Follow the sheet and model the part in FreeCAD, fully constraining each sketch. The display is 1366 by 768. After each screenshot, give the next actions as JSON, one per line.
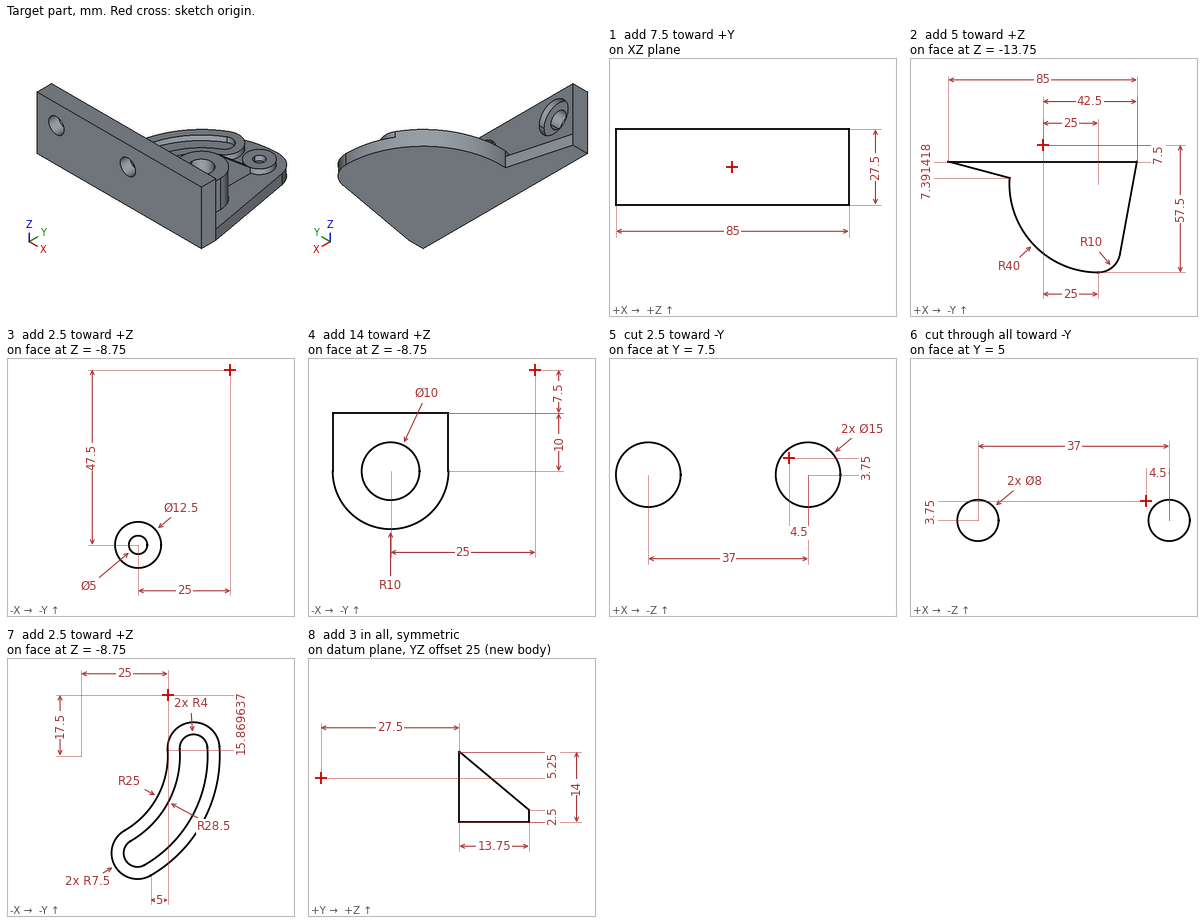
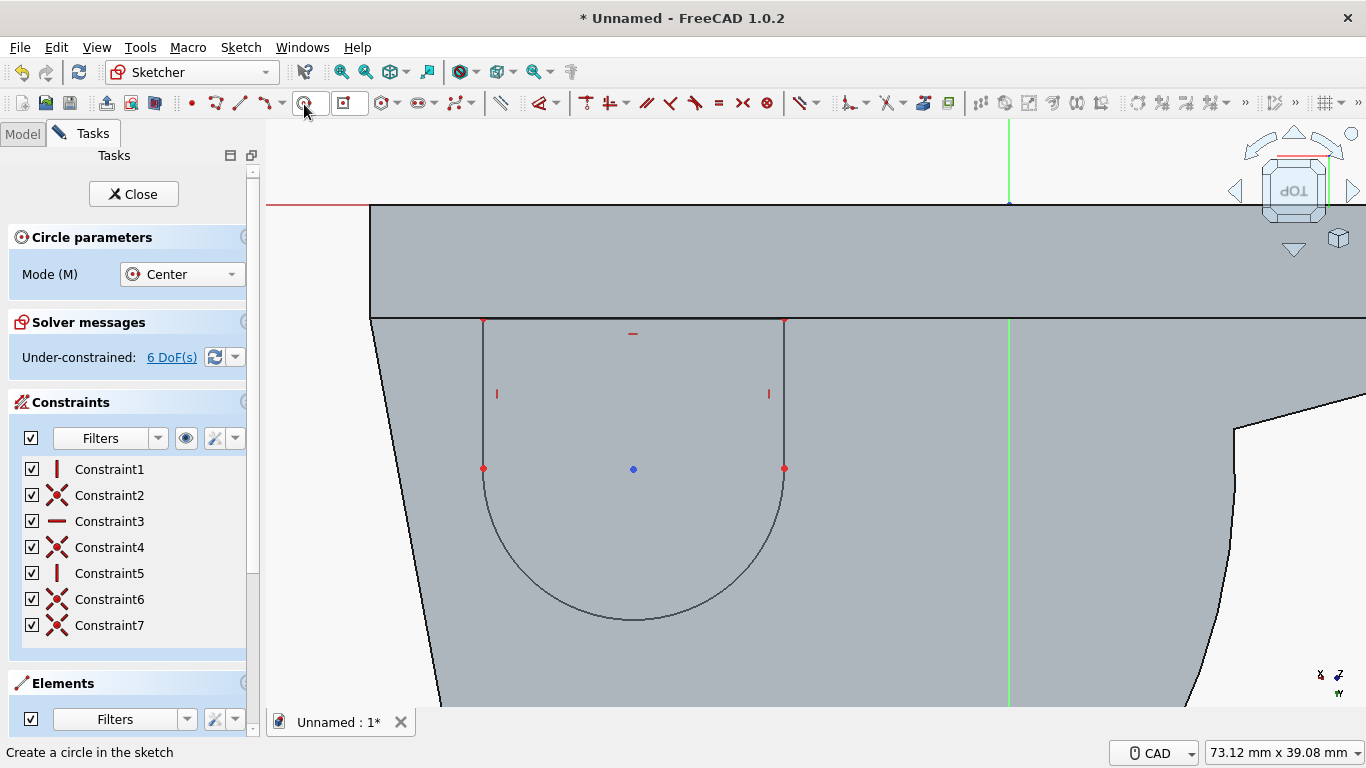
{"action": "left_click", "coordinate": [633, 468]}
{"action": "mouse_move", "coordinate": [687, 415]}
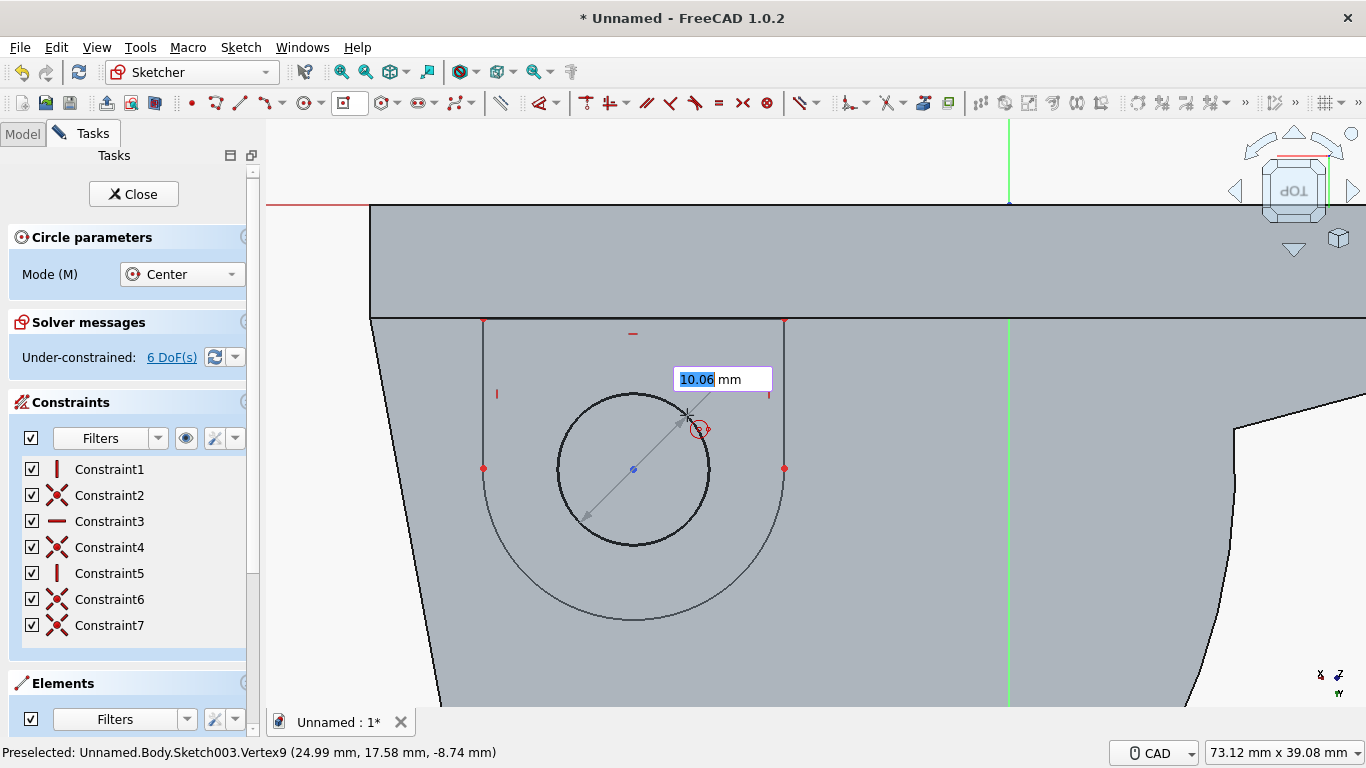
{"action": "type", "text": "10"}
{"action": "key", "text": "Return"}
{"action": "key", "text": "Escape"}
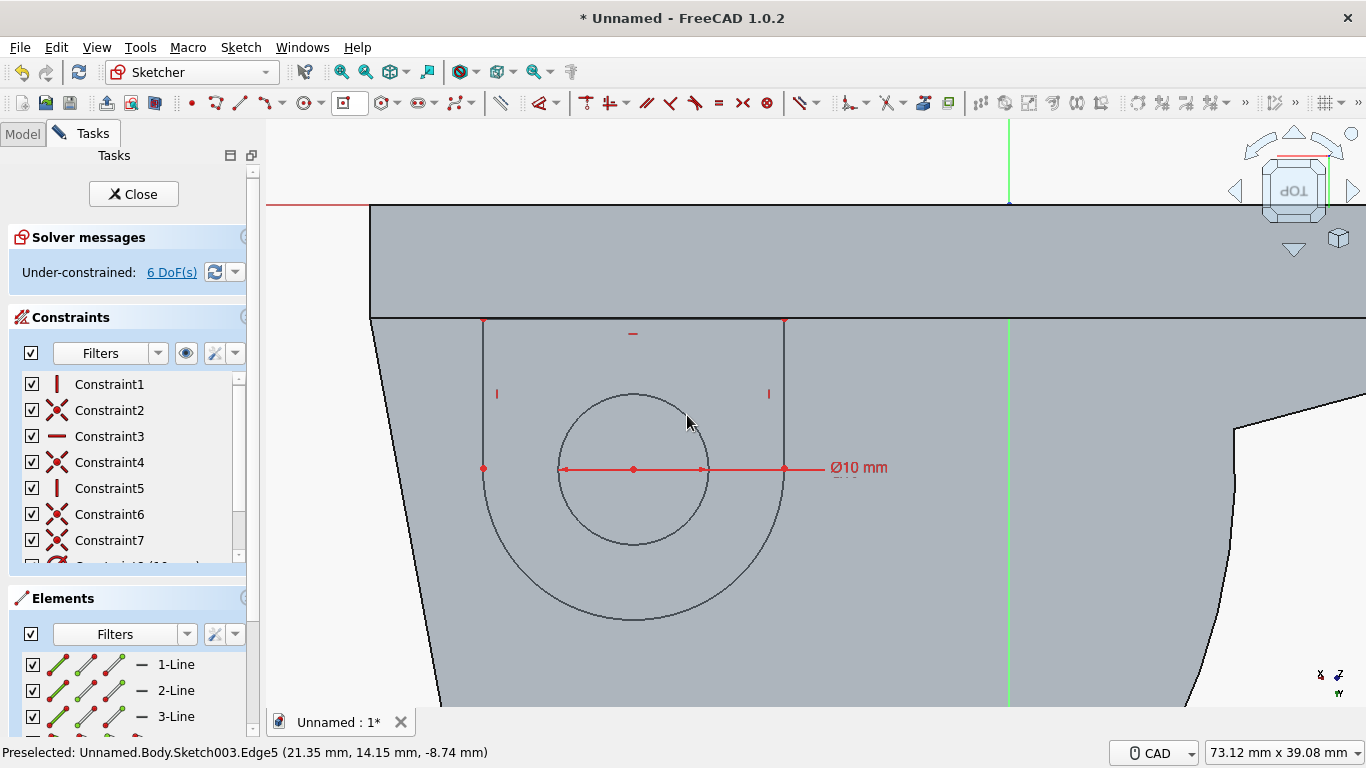
{"action": "left_click", "coordinate": [784, 424]}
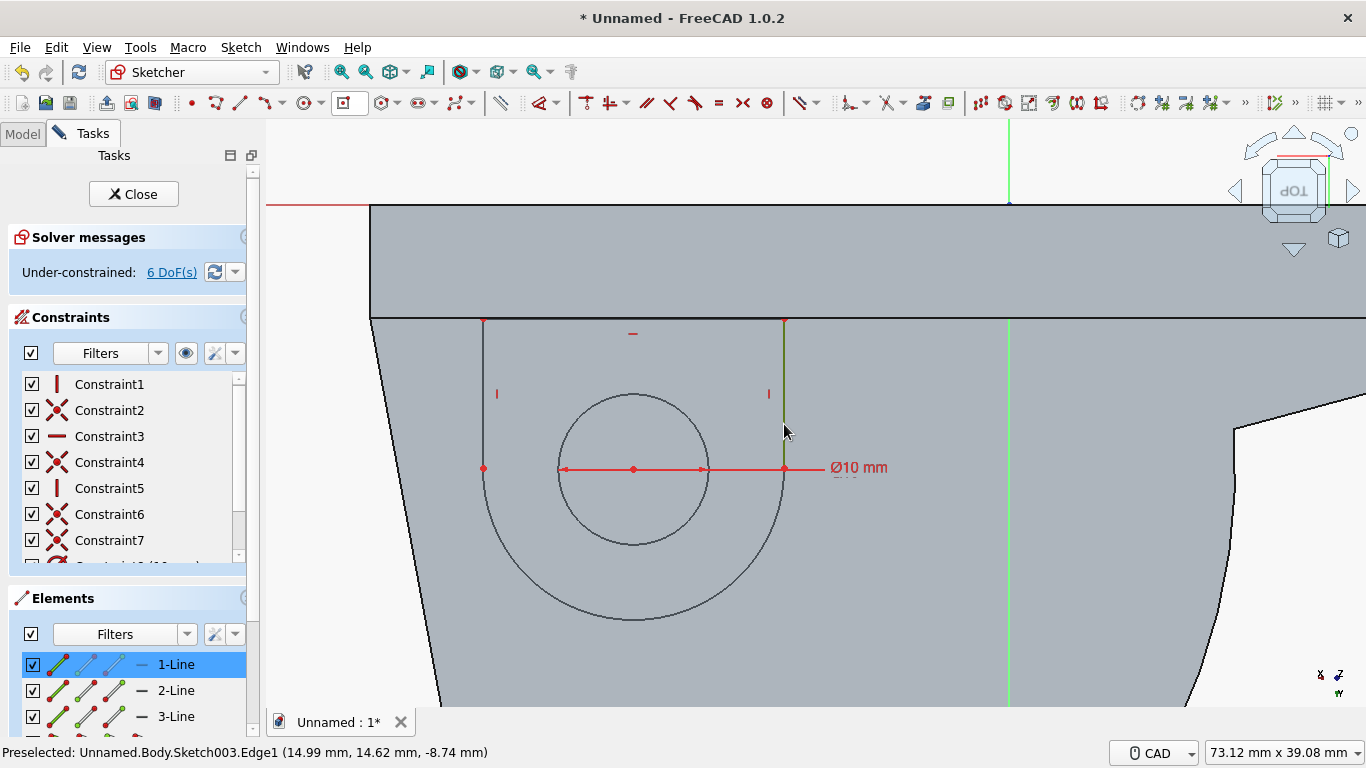
{"action": "left_click", "coordinate": [545, 591]}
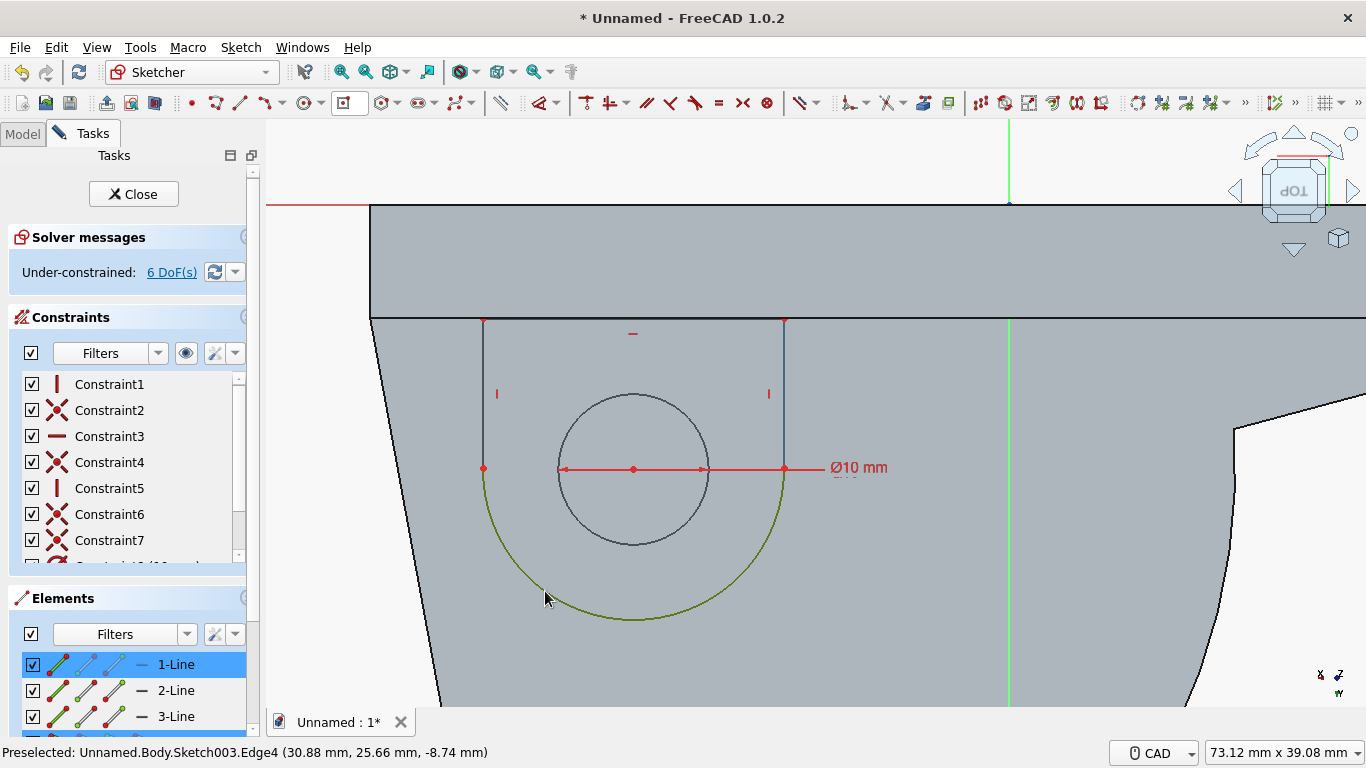
{"action": "left_click", "coordinate": [696, 104]}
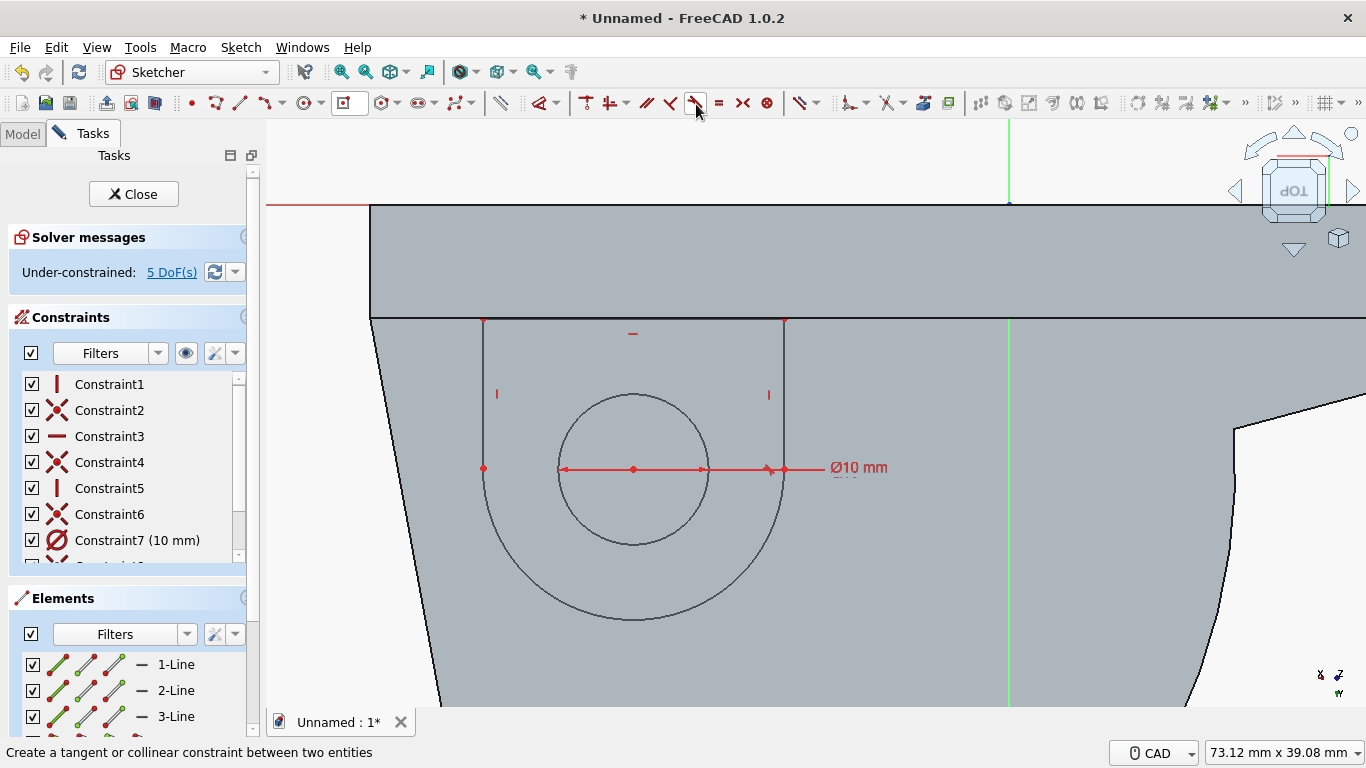
{"action": "left_click", "coordinate": [483, 364]}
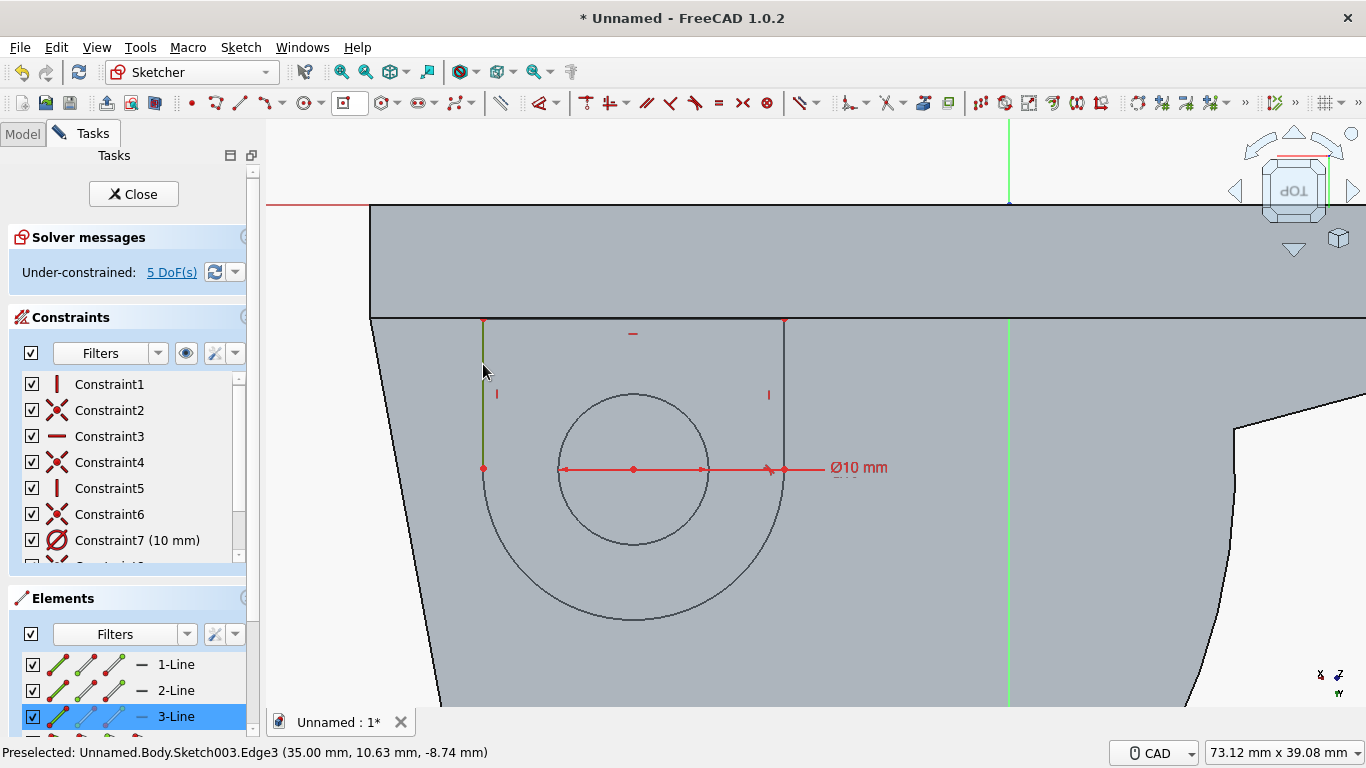
{"action": "left_click", "coordinate": [545, 591]}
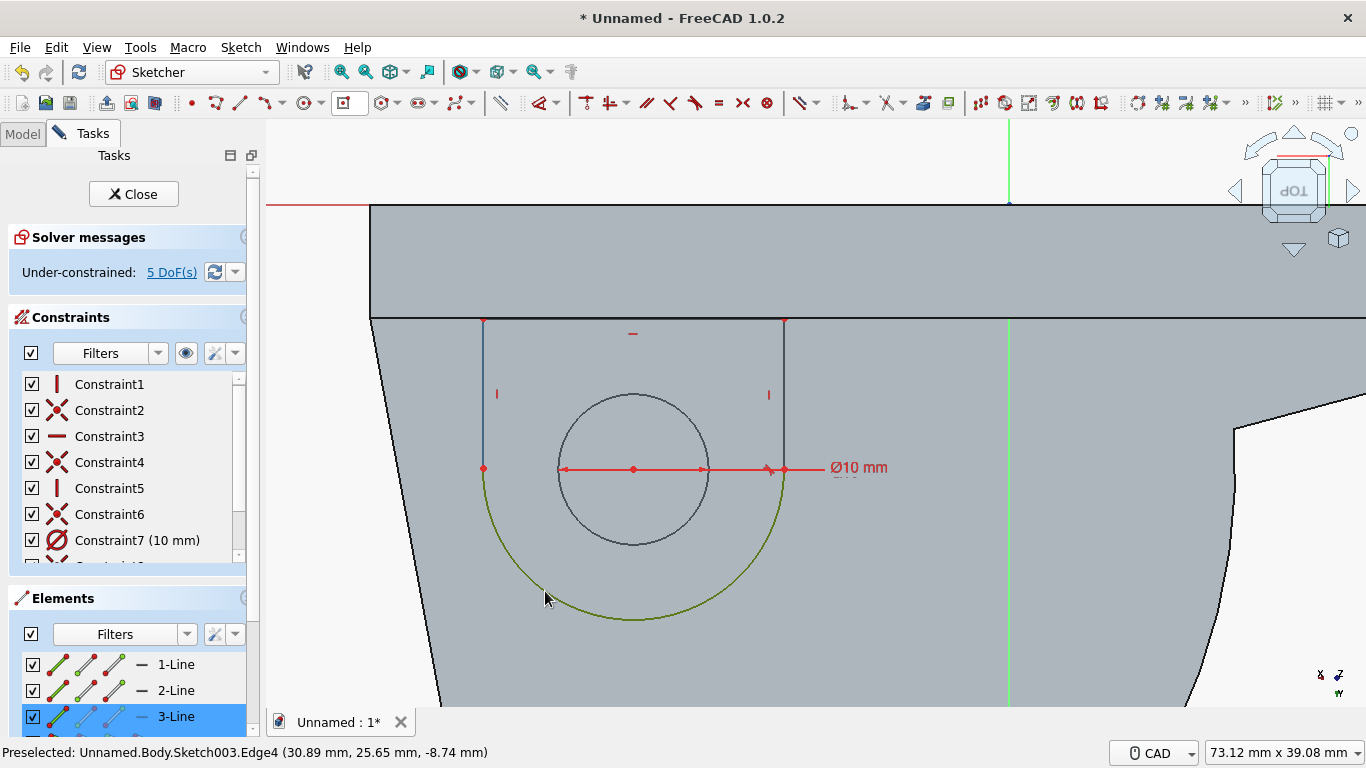
{"action": "left_click", "coordinate": [696, 104]}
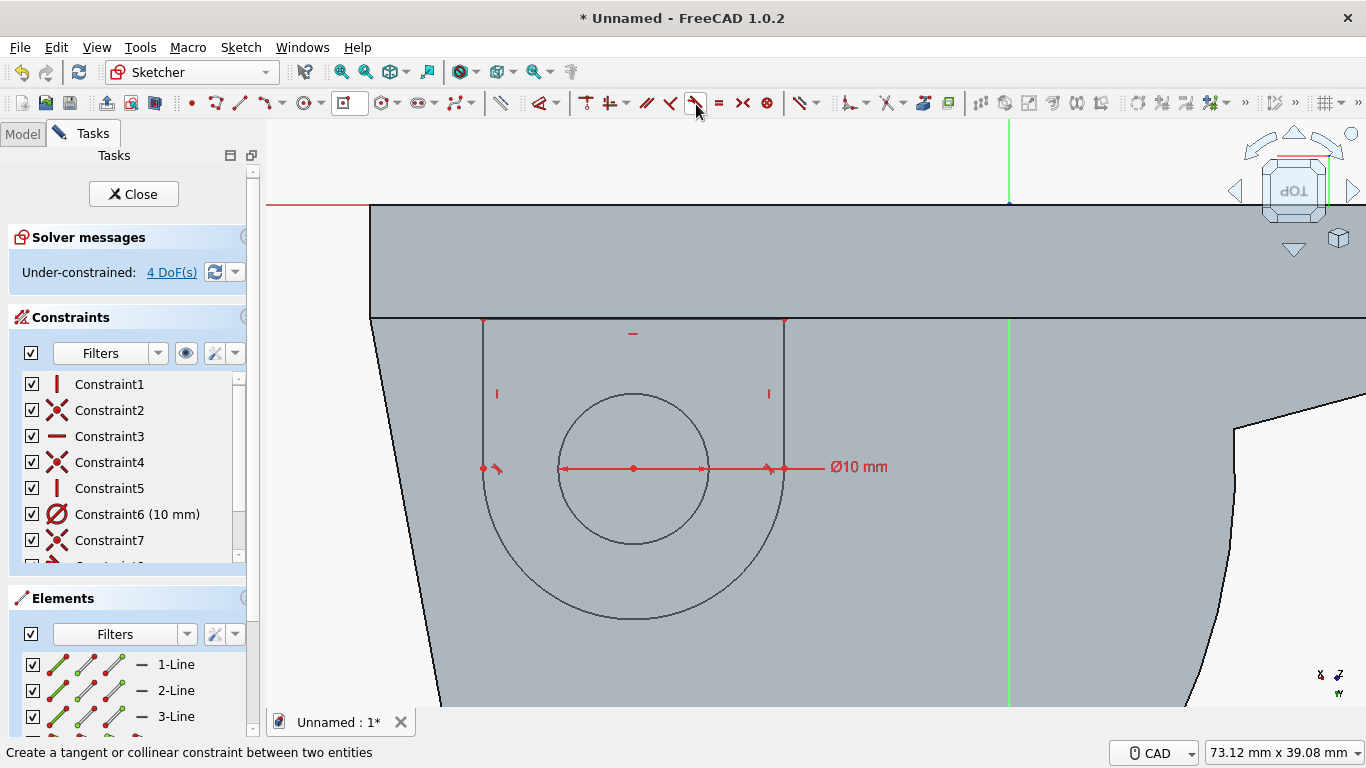
{"action": "left_click", "coordinate": [540, 104]}